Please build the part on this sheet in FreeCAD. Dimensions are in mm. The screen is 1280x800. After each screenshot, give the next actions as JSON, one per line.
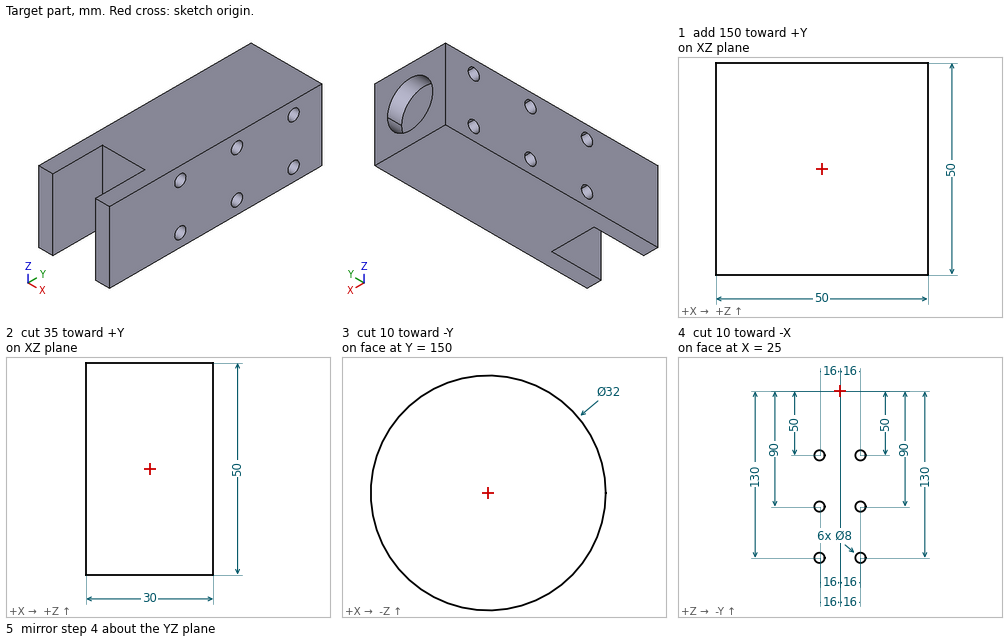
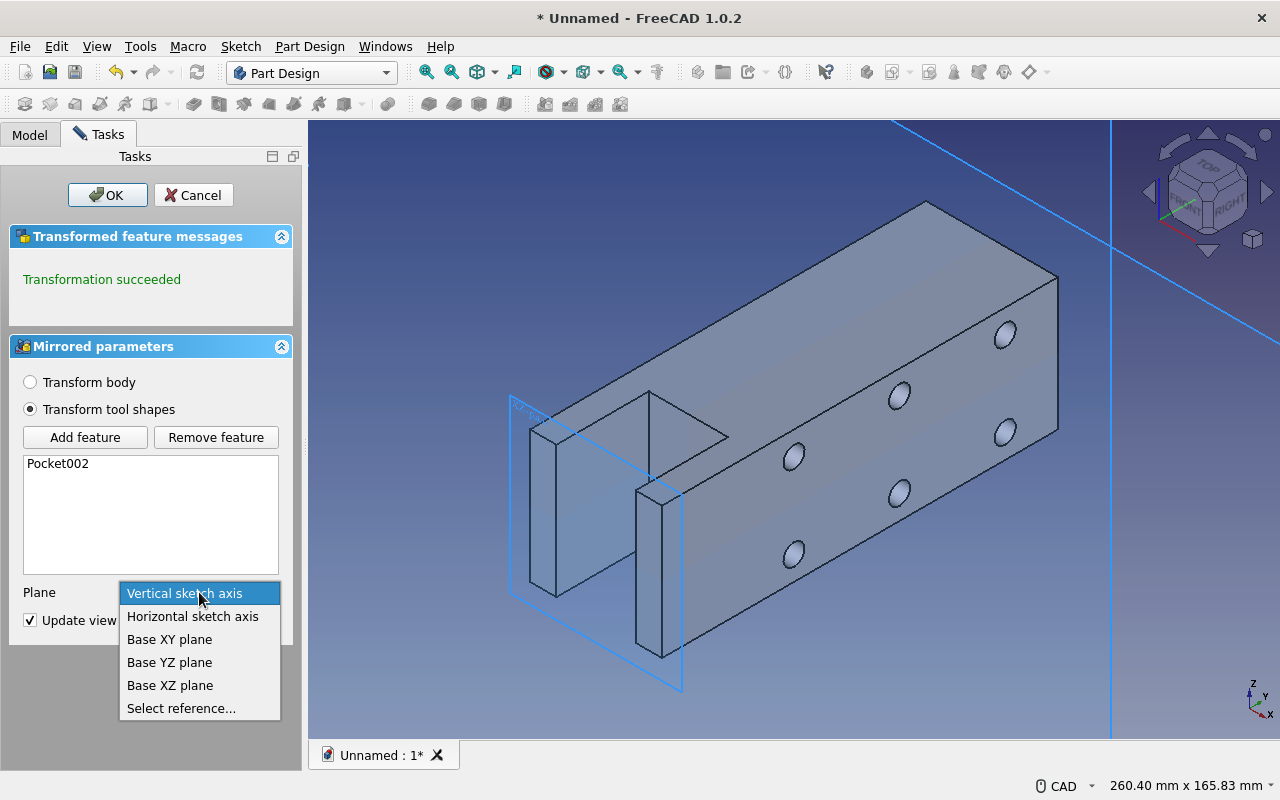
{"action": "left_click", "coordinate": [198, 662]}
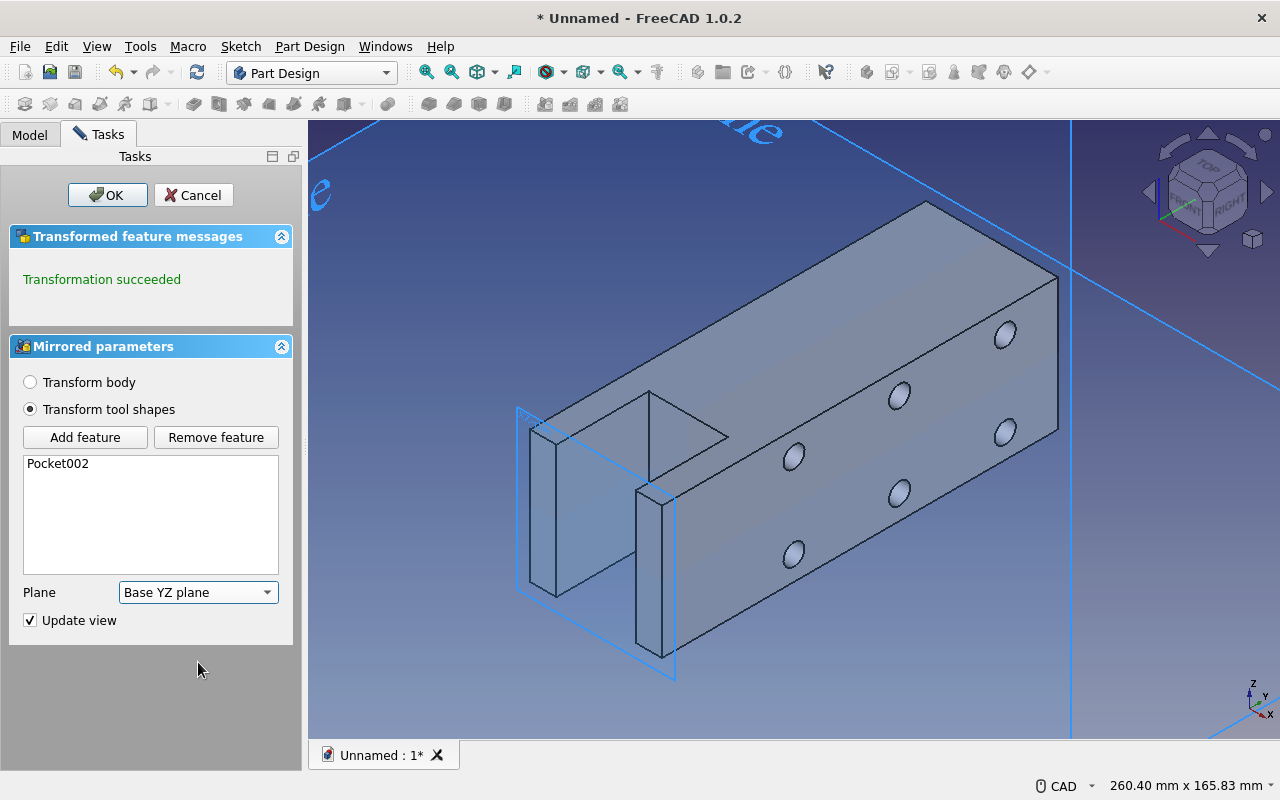
{"action": "left_click", "coordinate": [108, 195]}